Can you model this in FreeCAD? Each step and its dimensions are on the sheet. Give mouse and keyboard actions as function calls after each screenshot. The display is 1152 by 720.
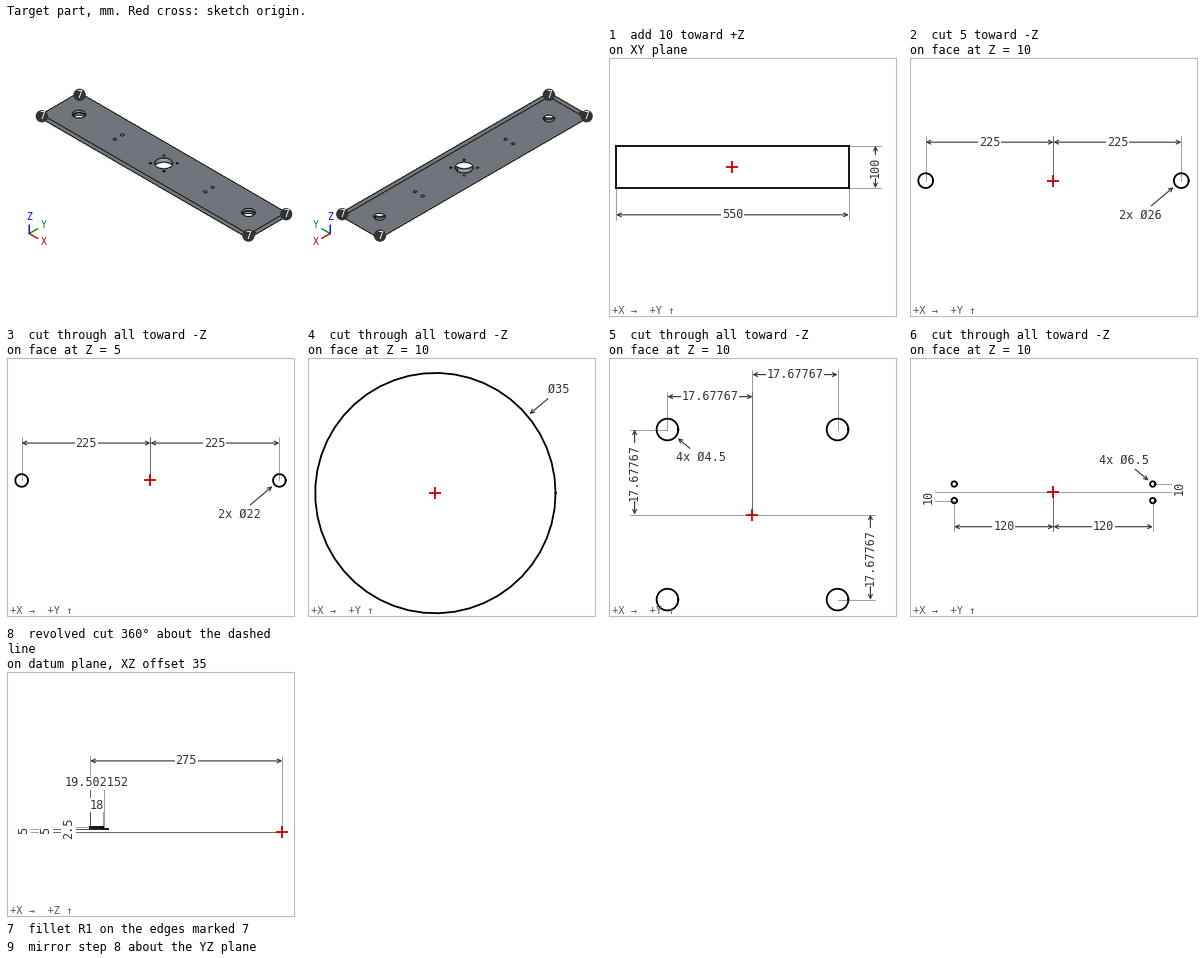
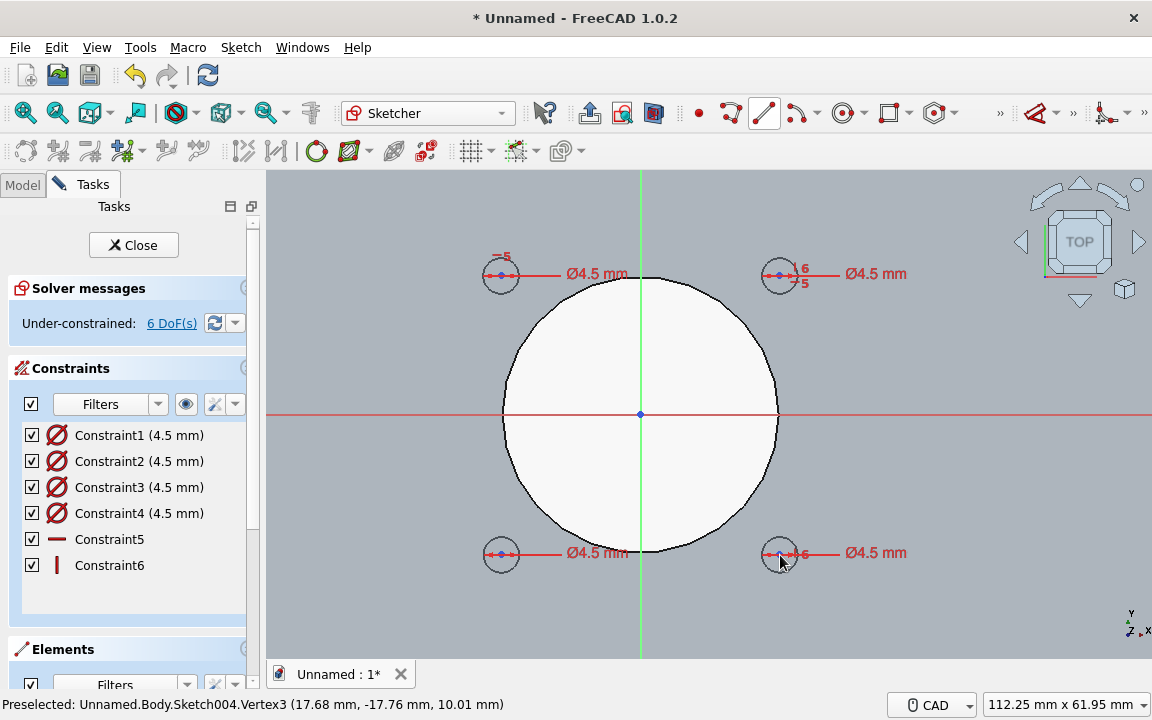
click(501, 276)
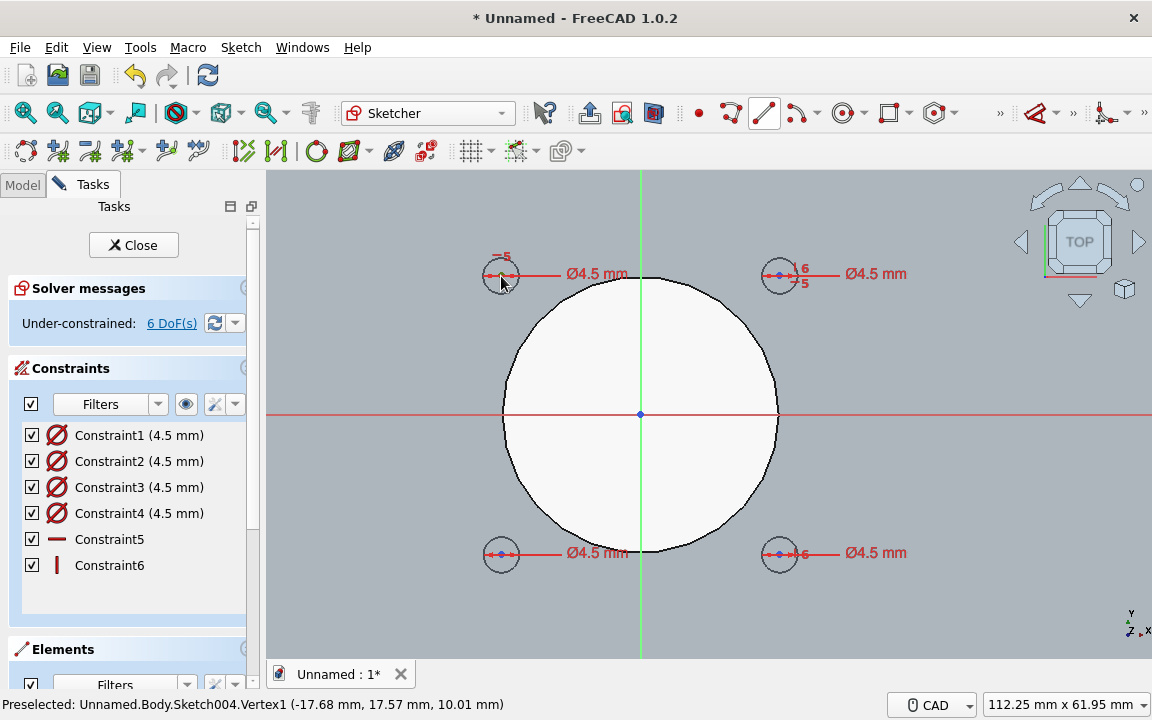
click(501, 555)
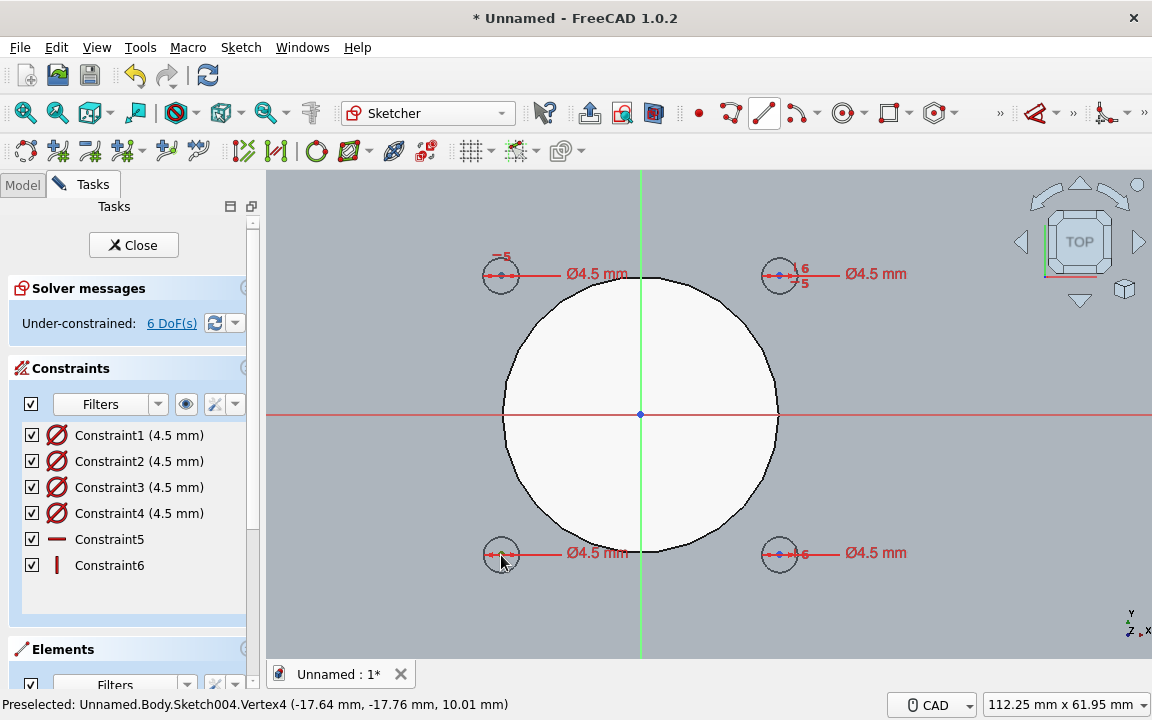
key(v)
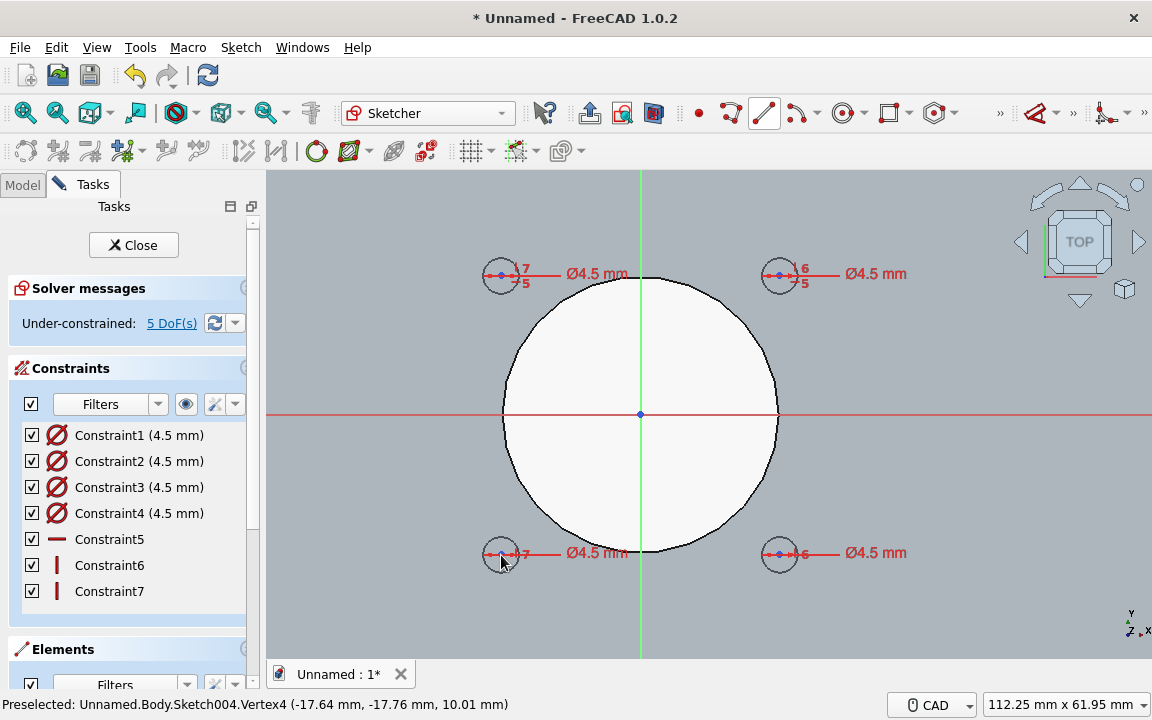
click(780, 555)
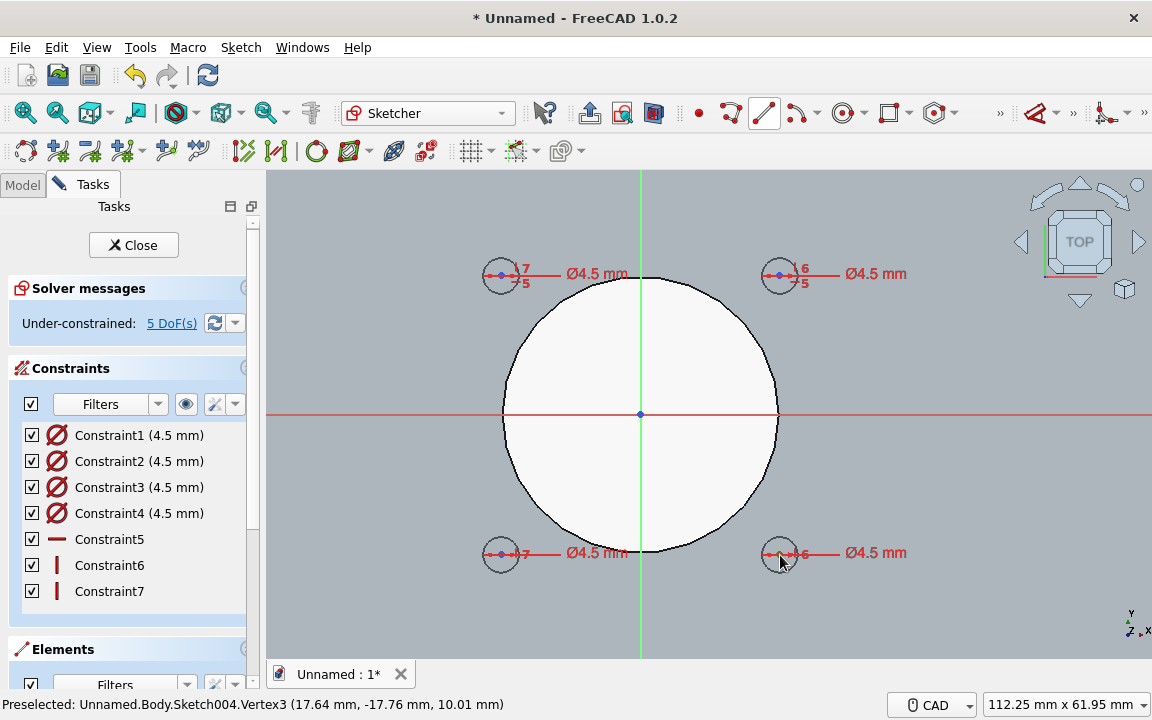
click(501, 555)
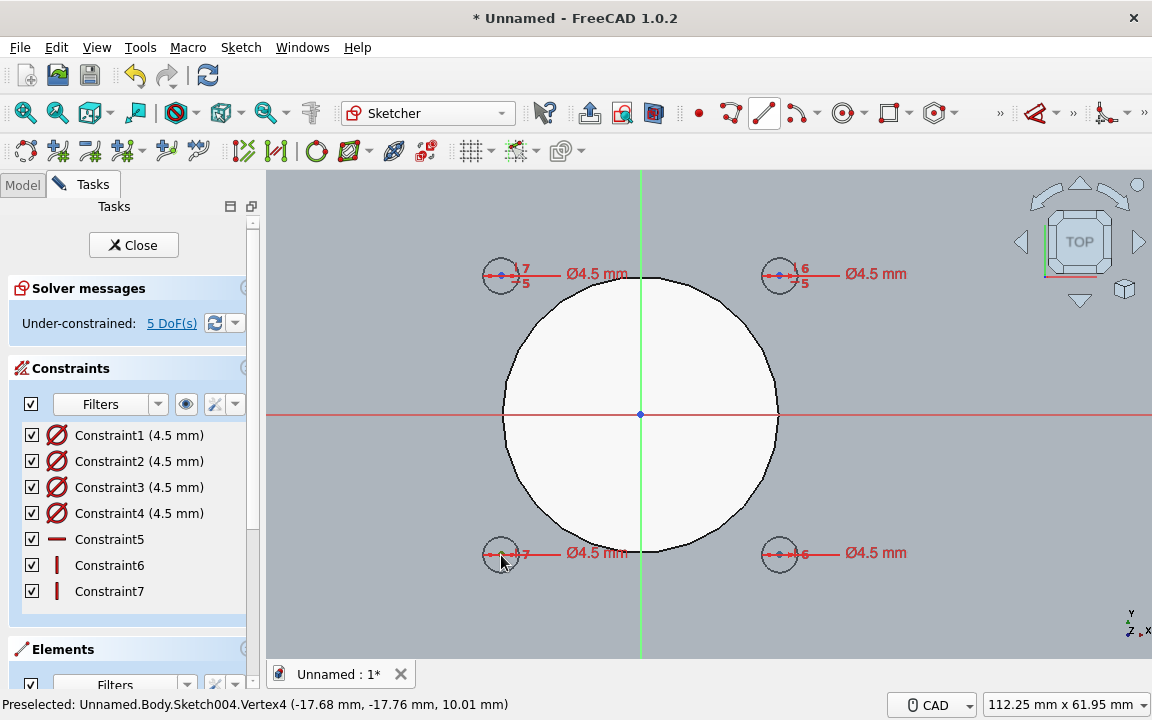
key(h)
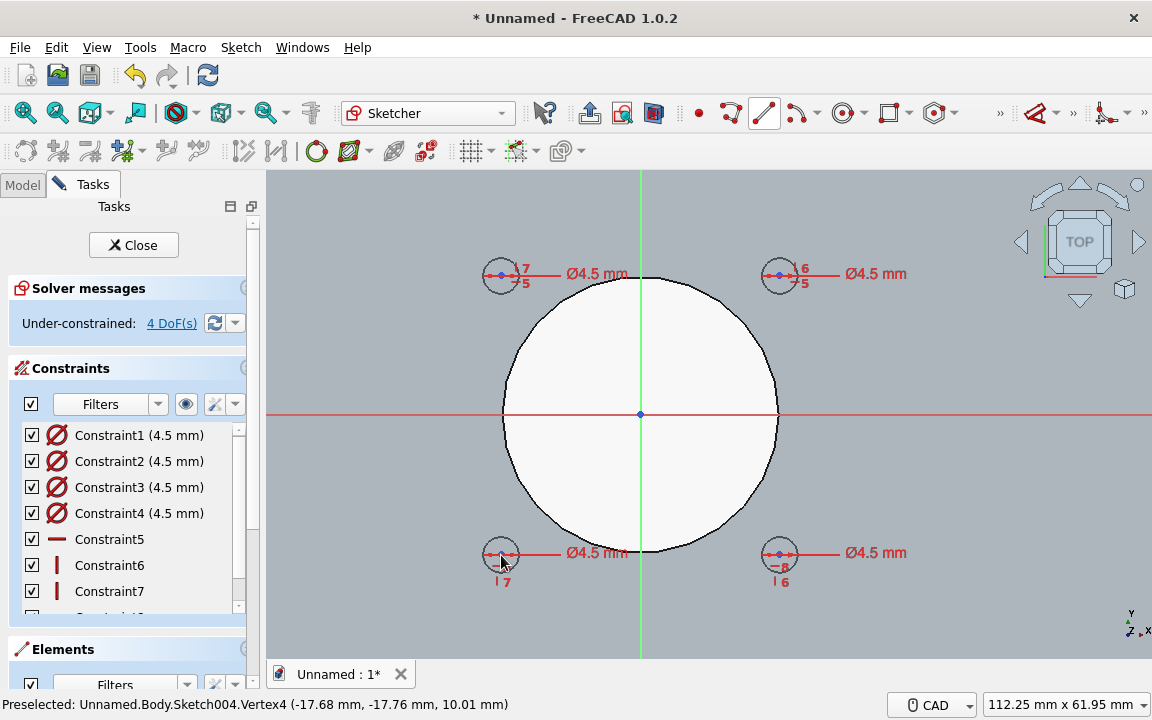
click(1036, 114)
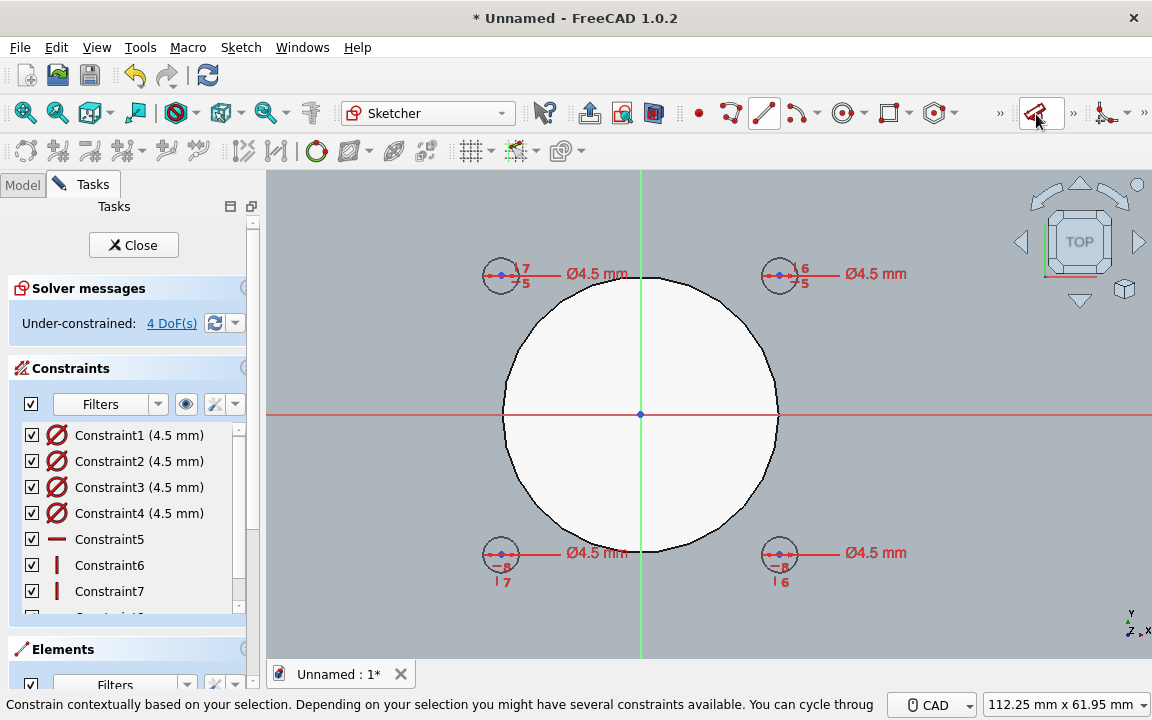
click(501, 276)
click(571, 242)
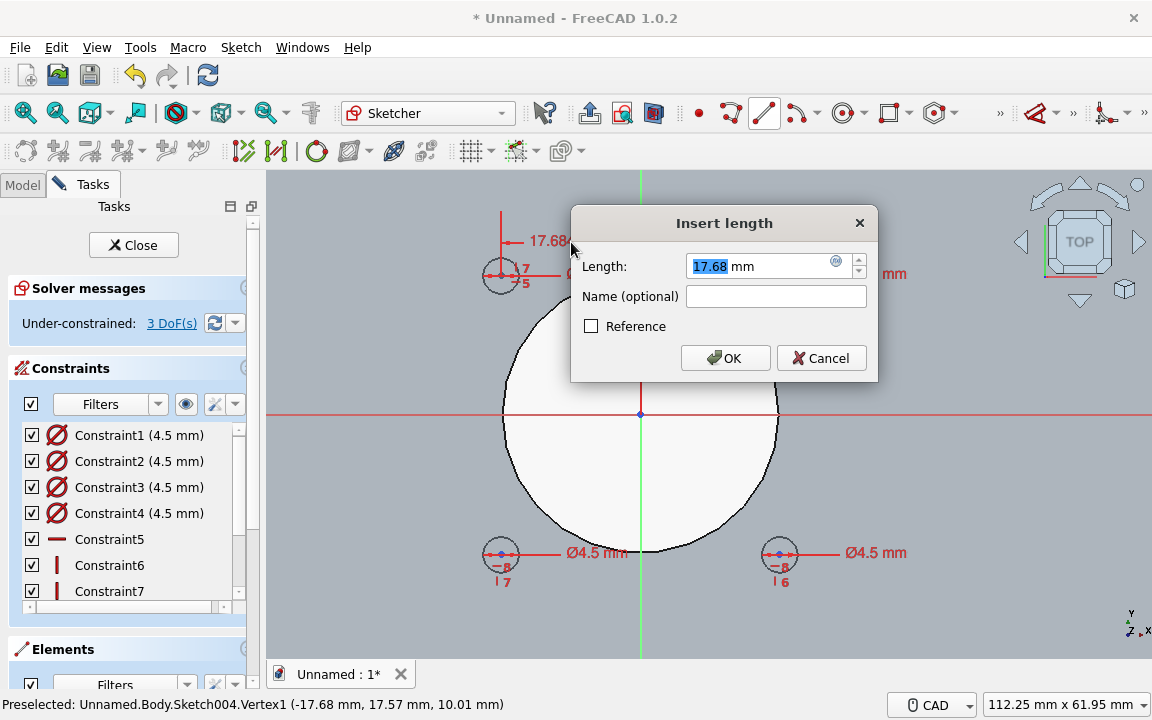
text(17.67767)
key(Return)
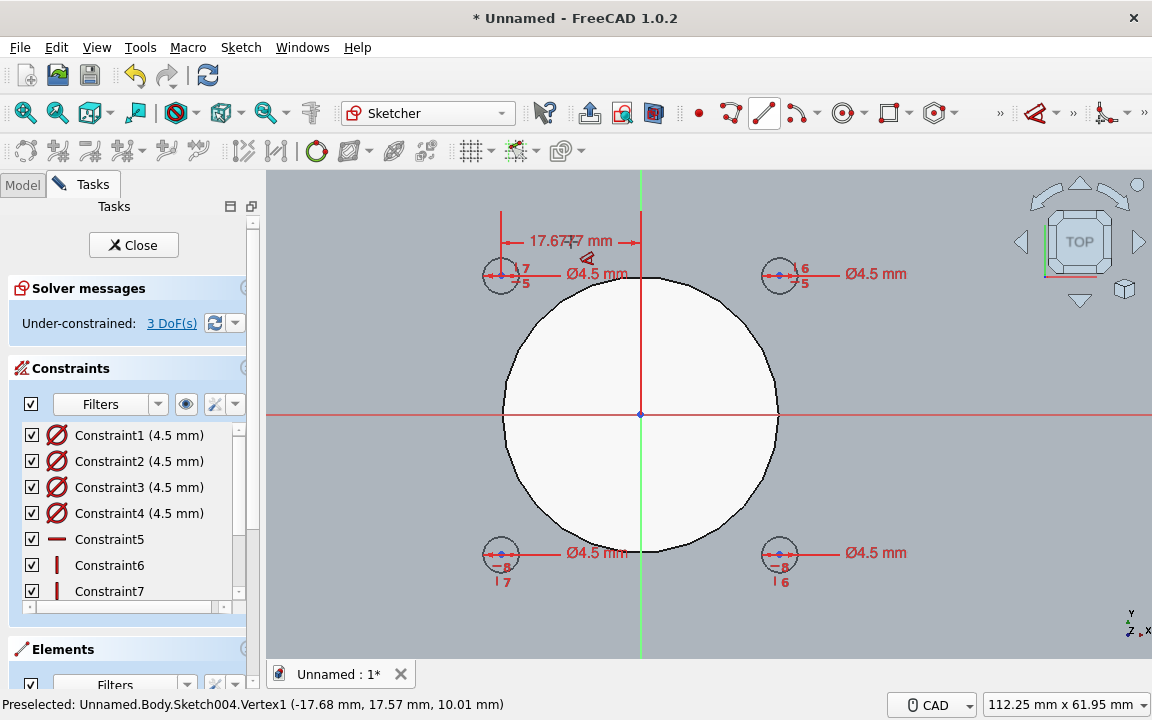
click(501, 276)
click(467, 345)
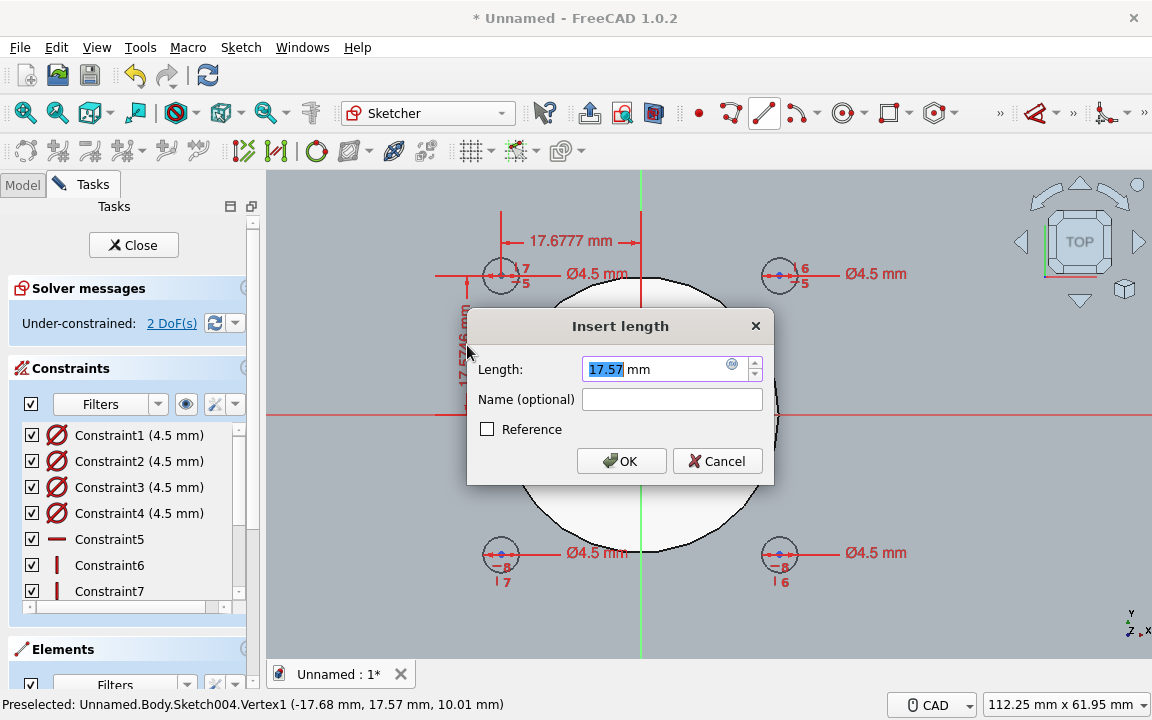
text(17.67767)
key(Return)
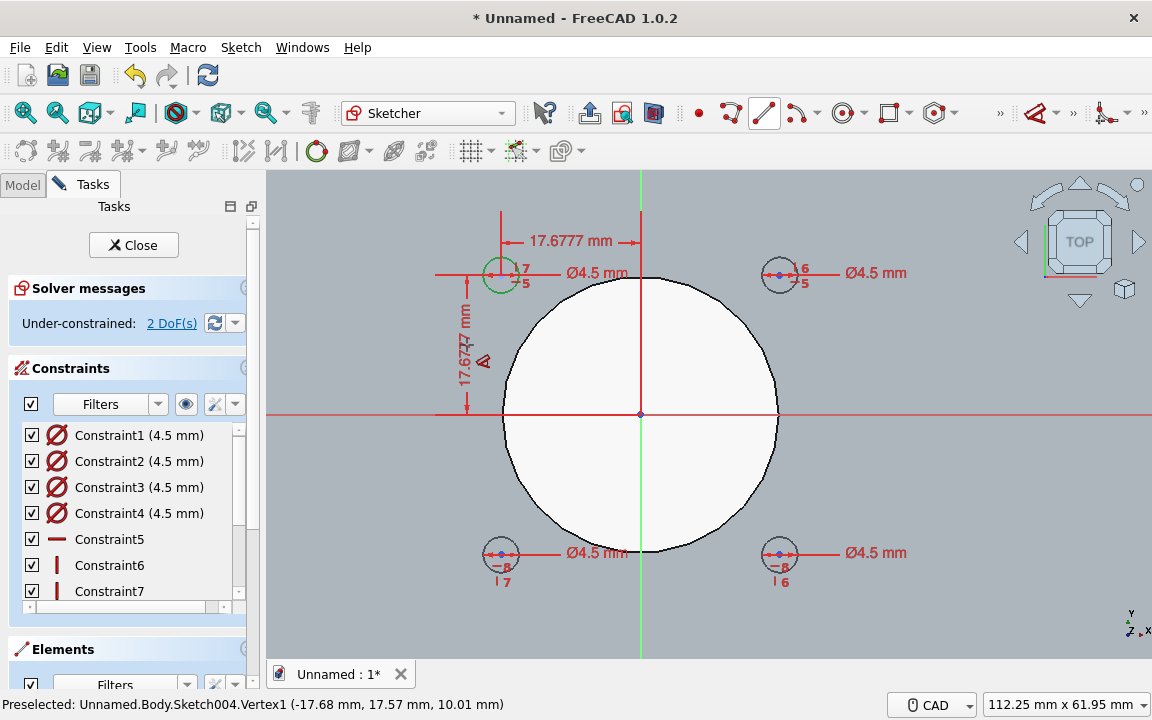
click(780, 275)
click(710, 241)